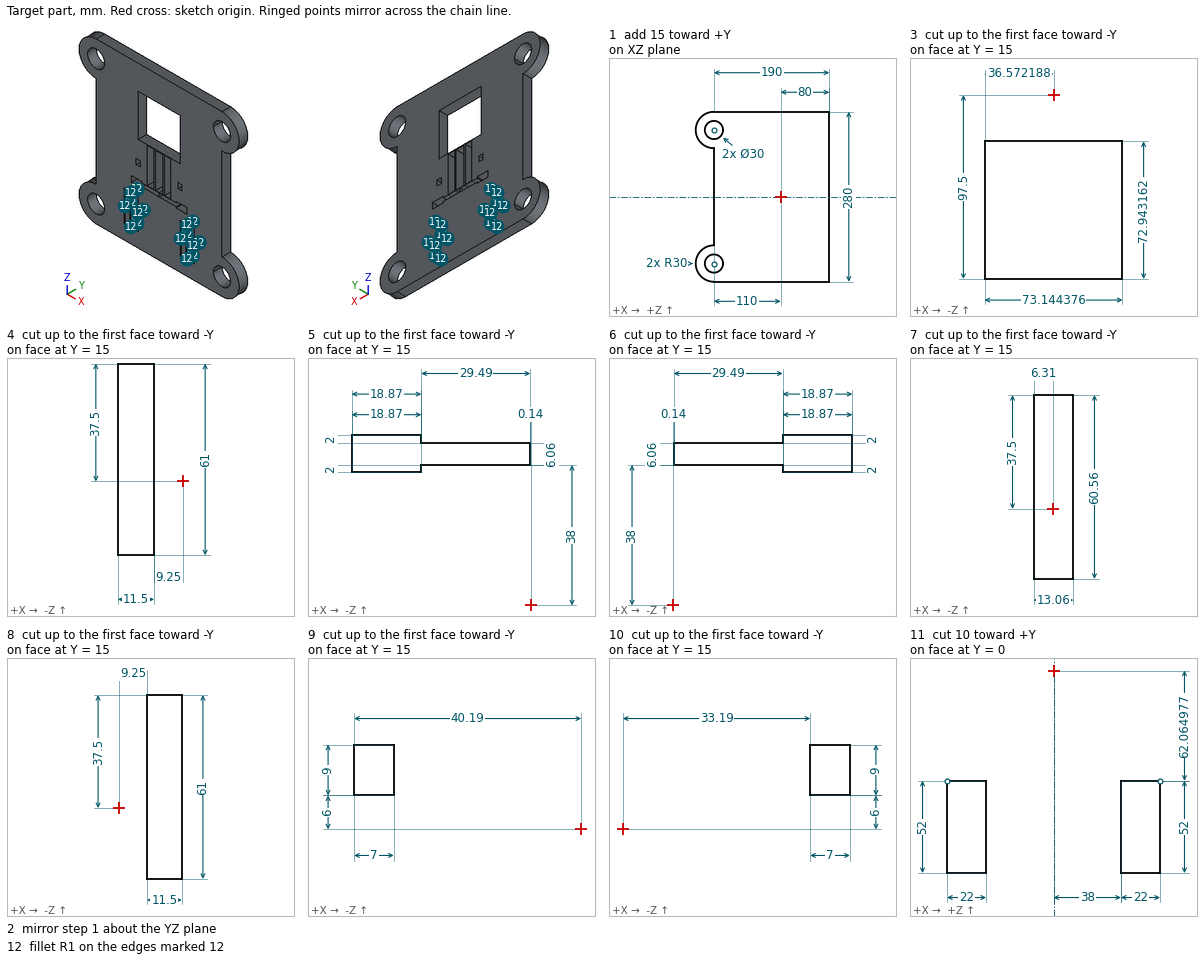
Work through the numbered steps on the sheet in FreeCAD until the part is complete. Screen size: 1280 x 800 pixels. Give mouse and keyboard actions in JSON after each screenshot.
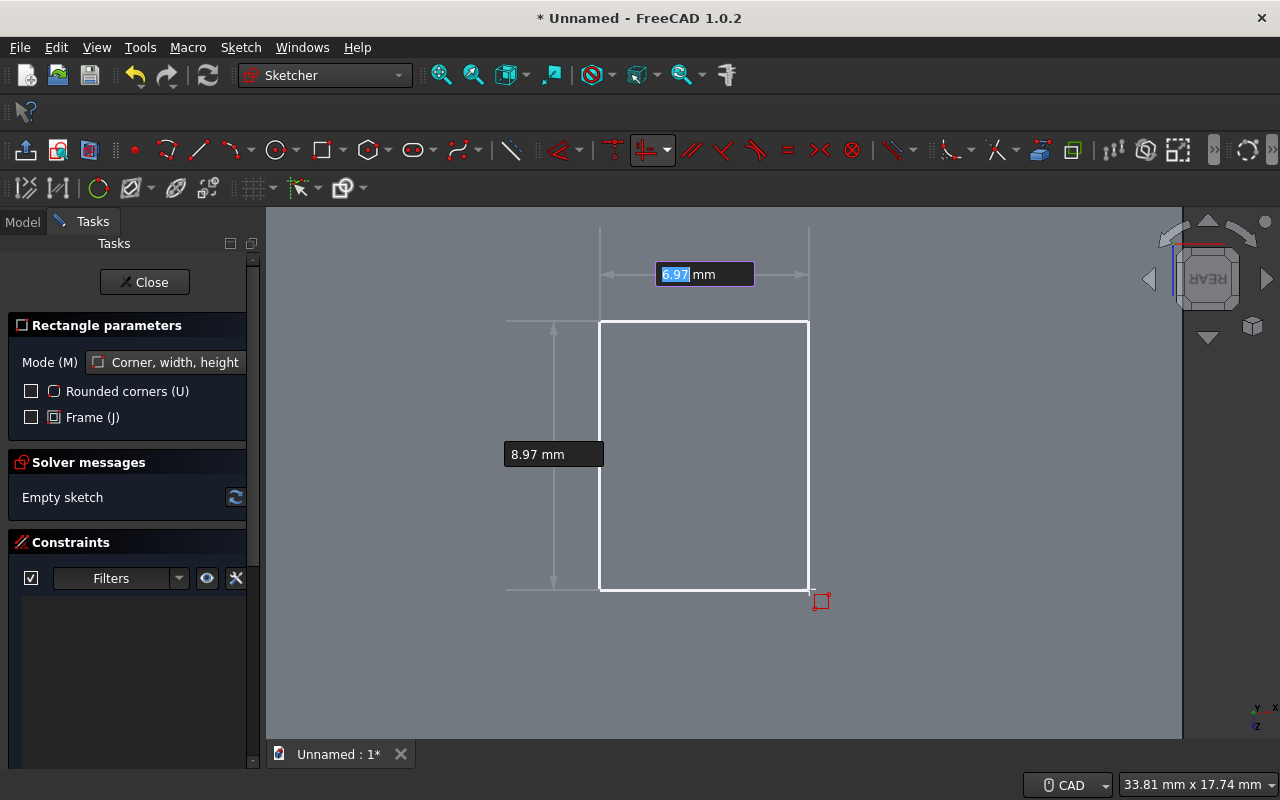
{"action": "type", "text": "7"}
{"action": "key", "text": "Tab"}
{"action": "type", "text": "9"}
{"action": "key", "text": "Return"}
{"action": "key", "text": "Escape"}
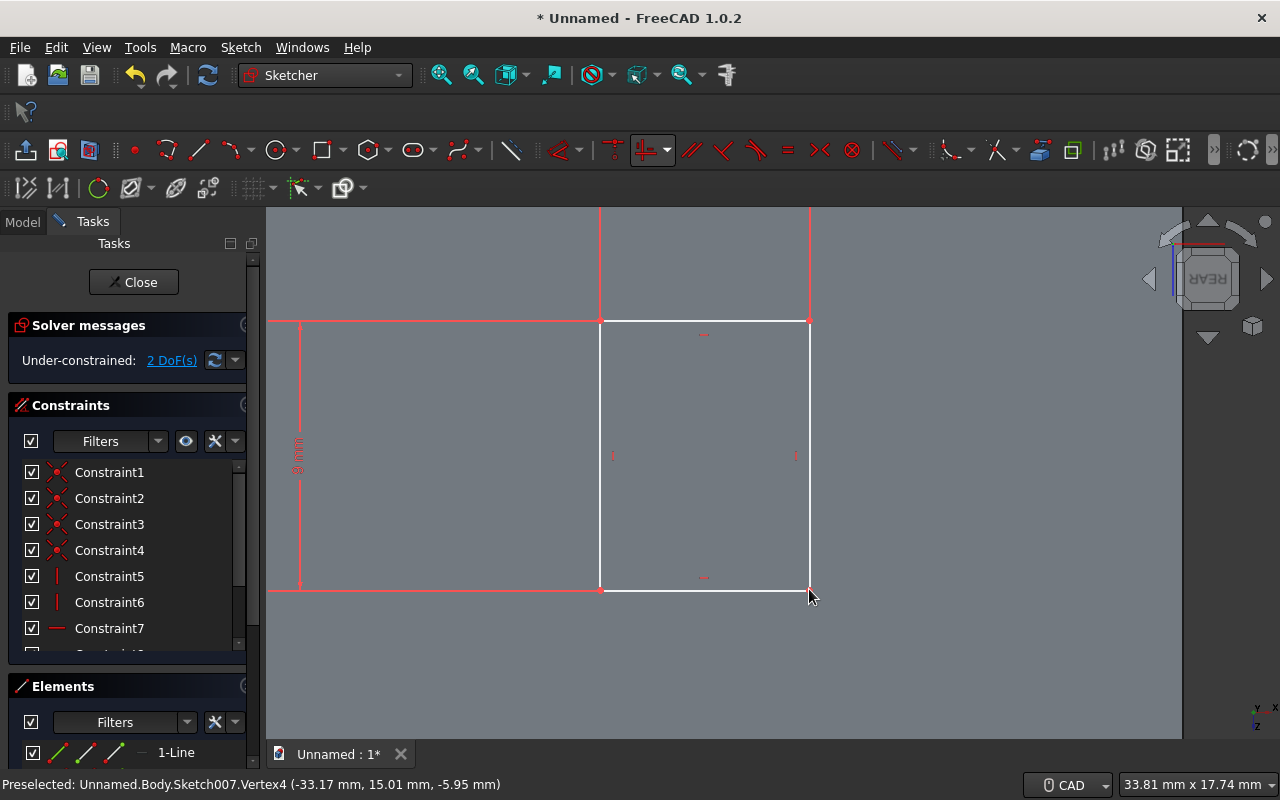
{"action": "left_click", "coordinate": [558, 150]}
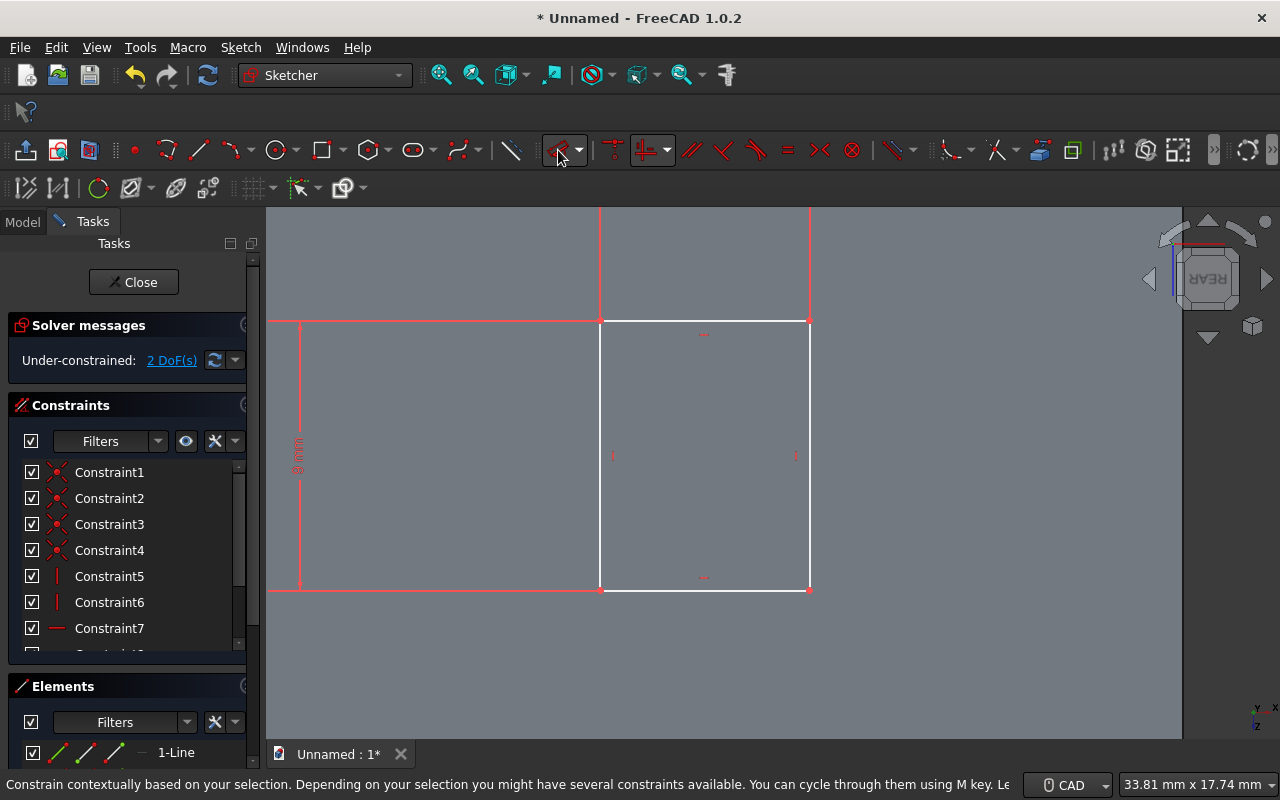
{"action": "left_click", "coordinate": [600, 591]}
{"action": "left_click", "coordinate": [566, 651]}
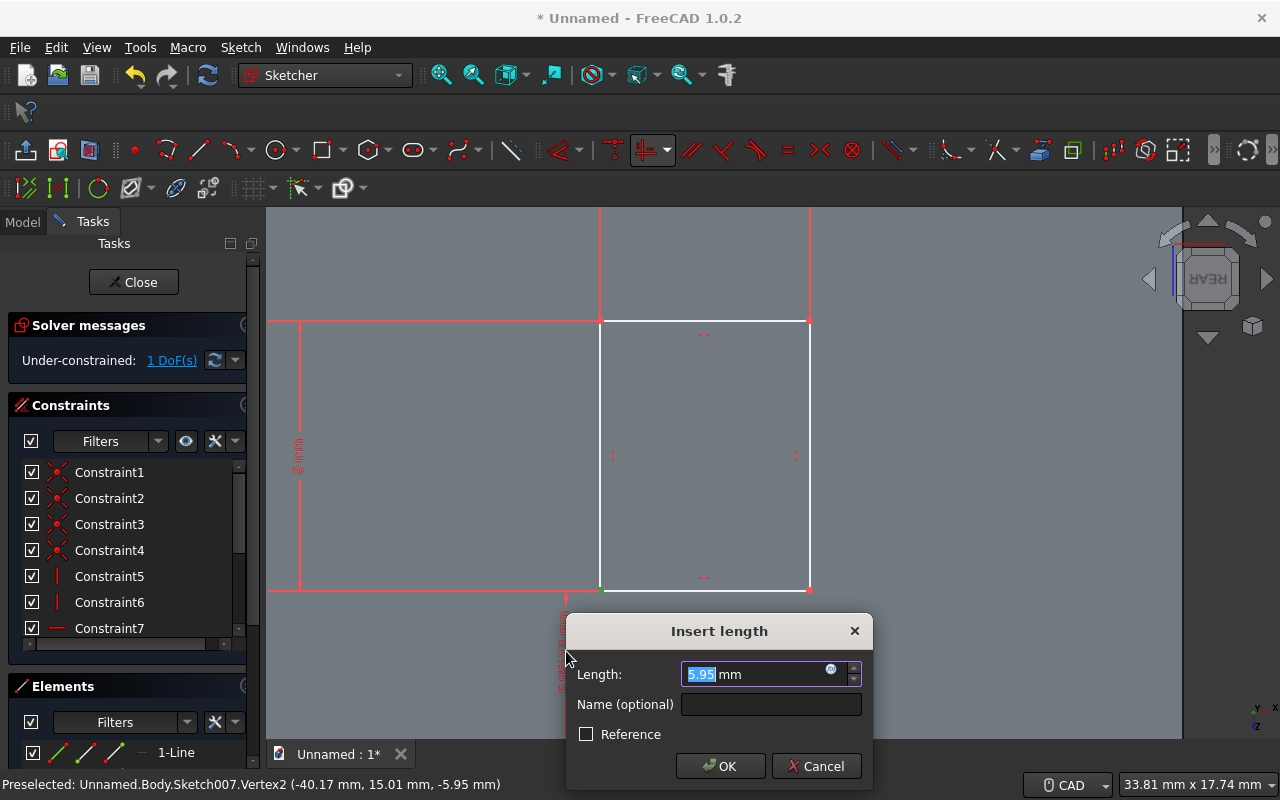
{"action": "type", "text": "6"}
{"action": "key", "text": "Return"}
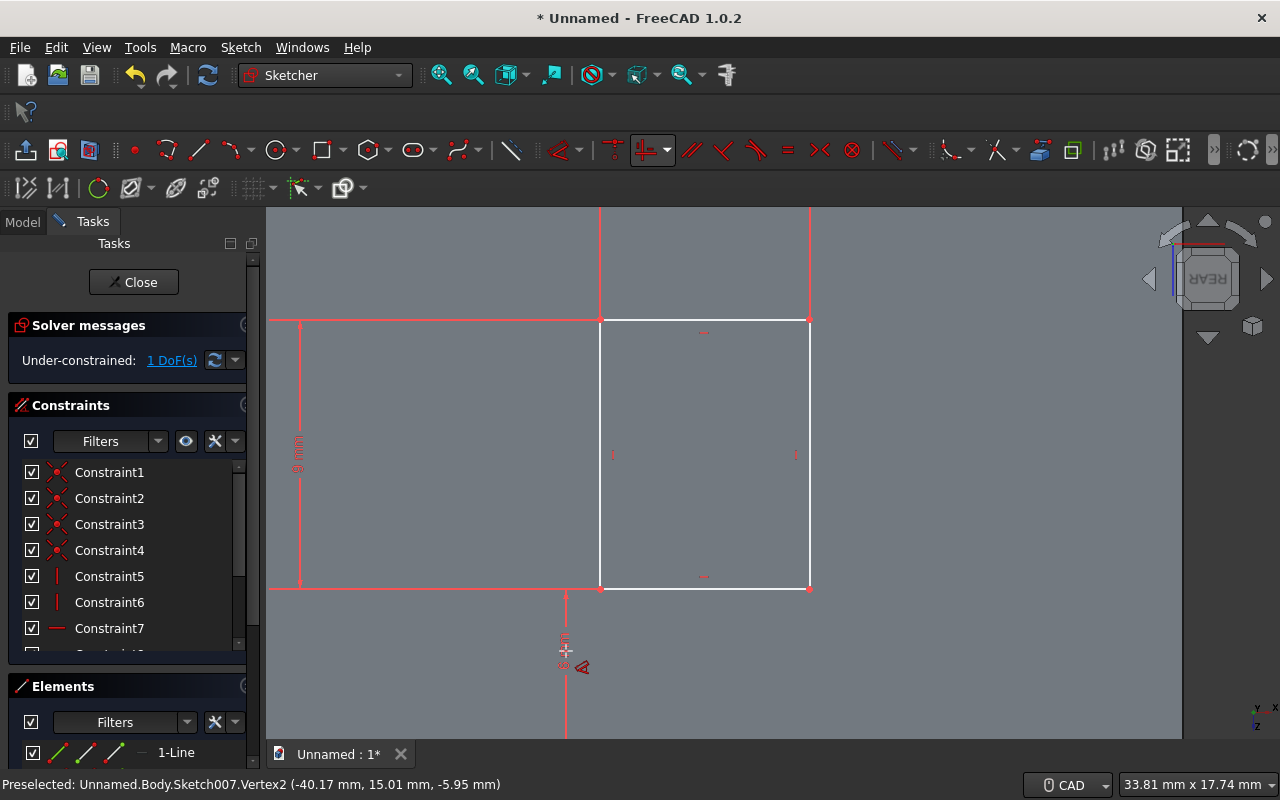
{"action": "left_click", "coordinate": [600, 320]}
{"action": "left_click", "coordinate": [858, 286]}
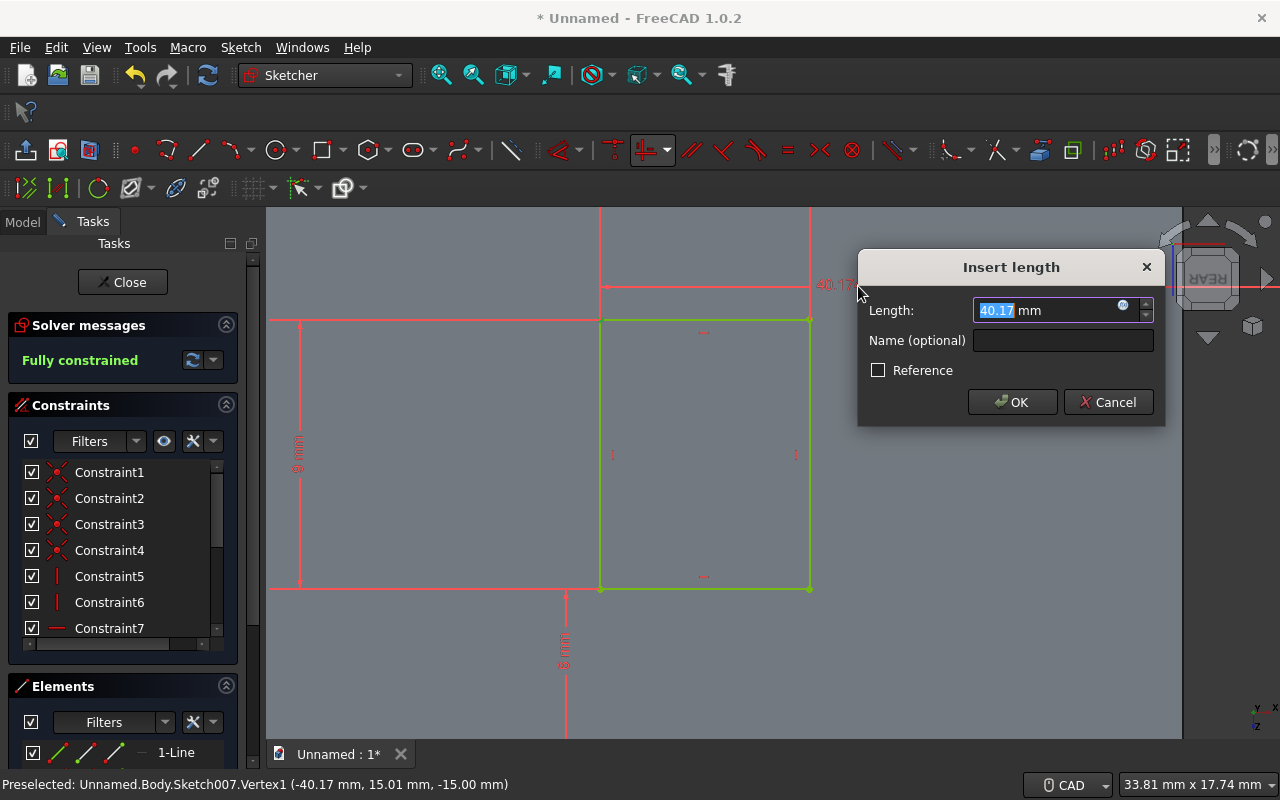
{"action": "type", "text": "40.19"}
{"action": "key", "text": "Return"}
{"action": "key", "text": "Escape"}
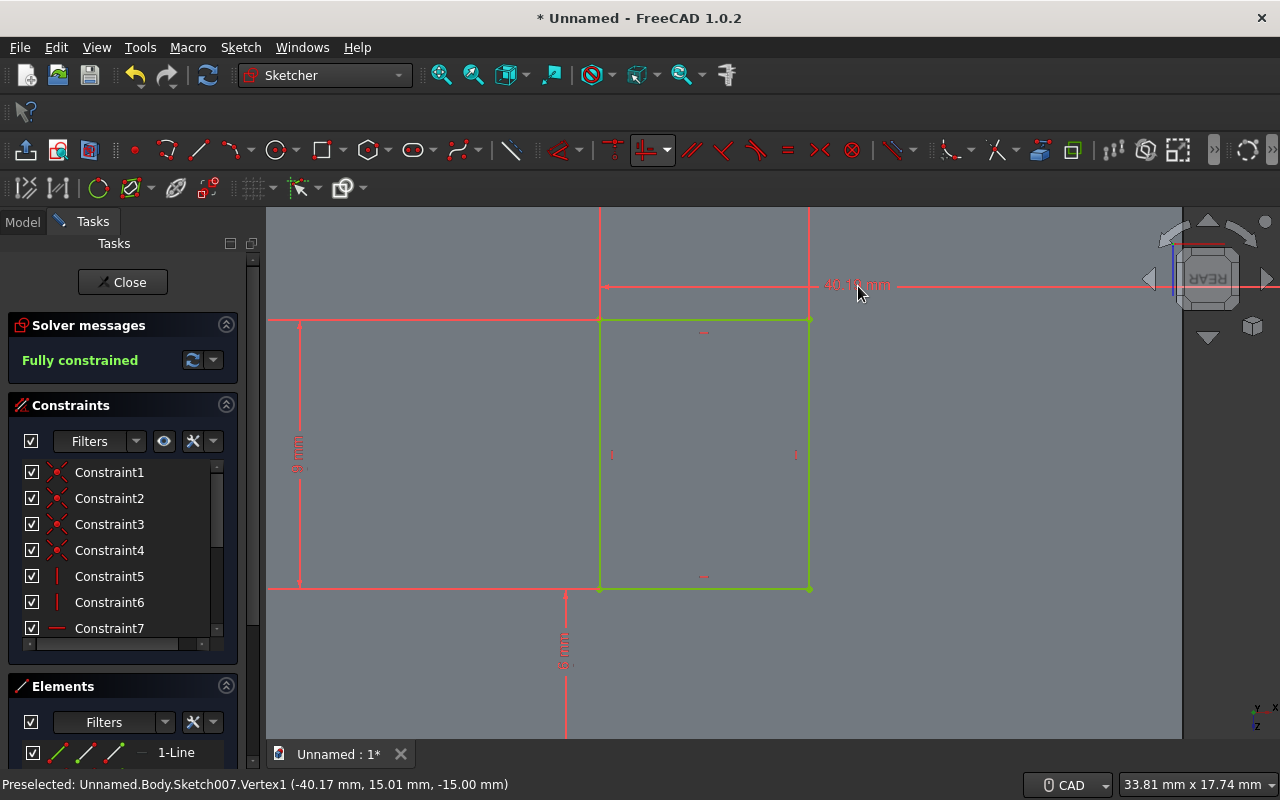
{"action": "left_click", "coordinate": [123, 282]}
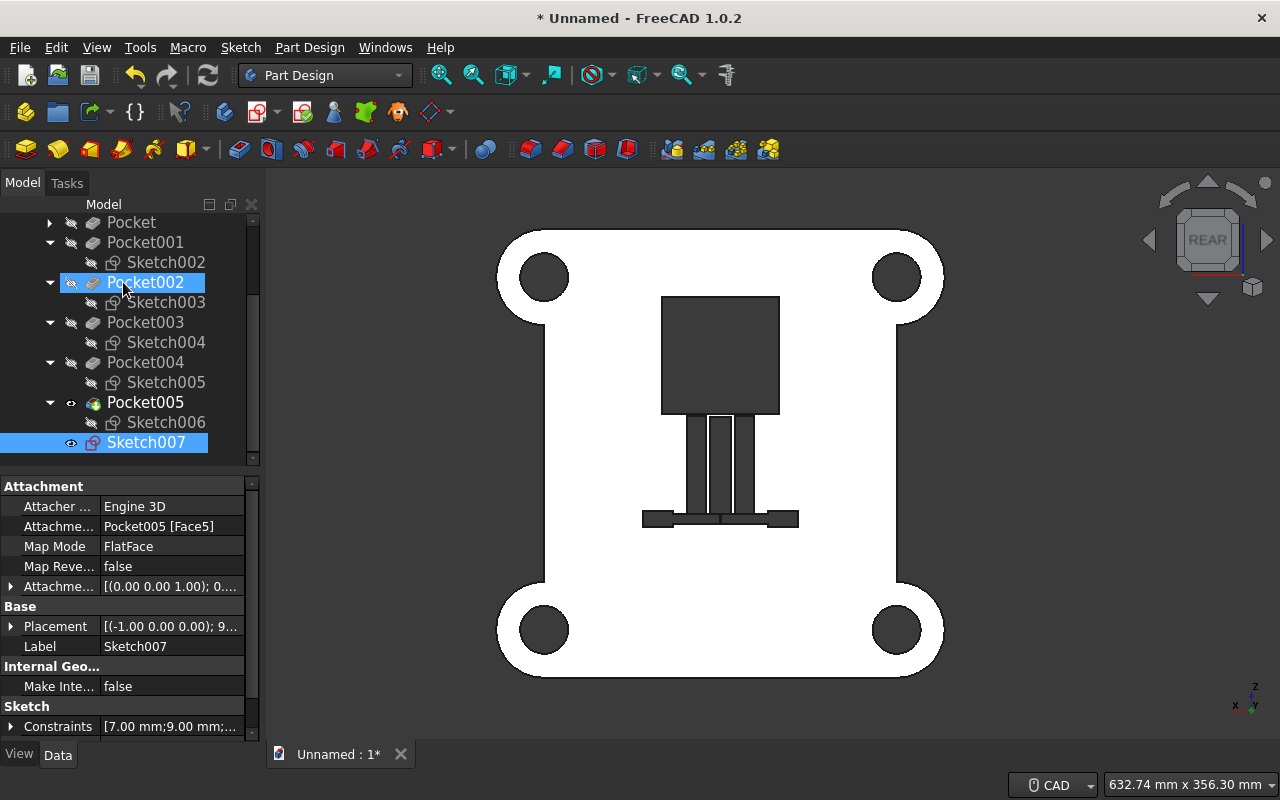
{"action": "left_click", "coordinate": [240, 150]}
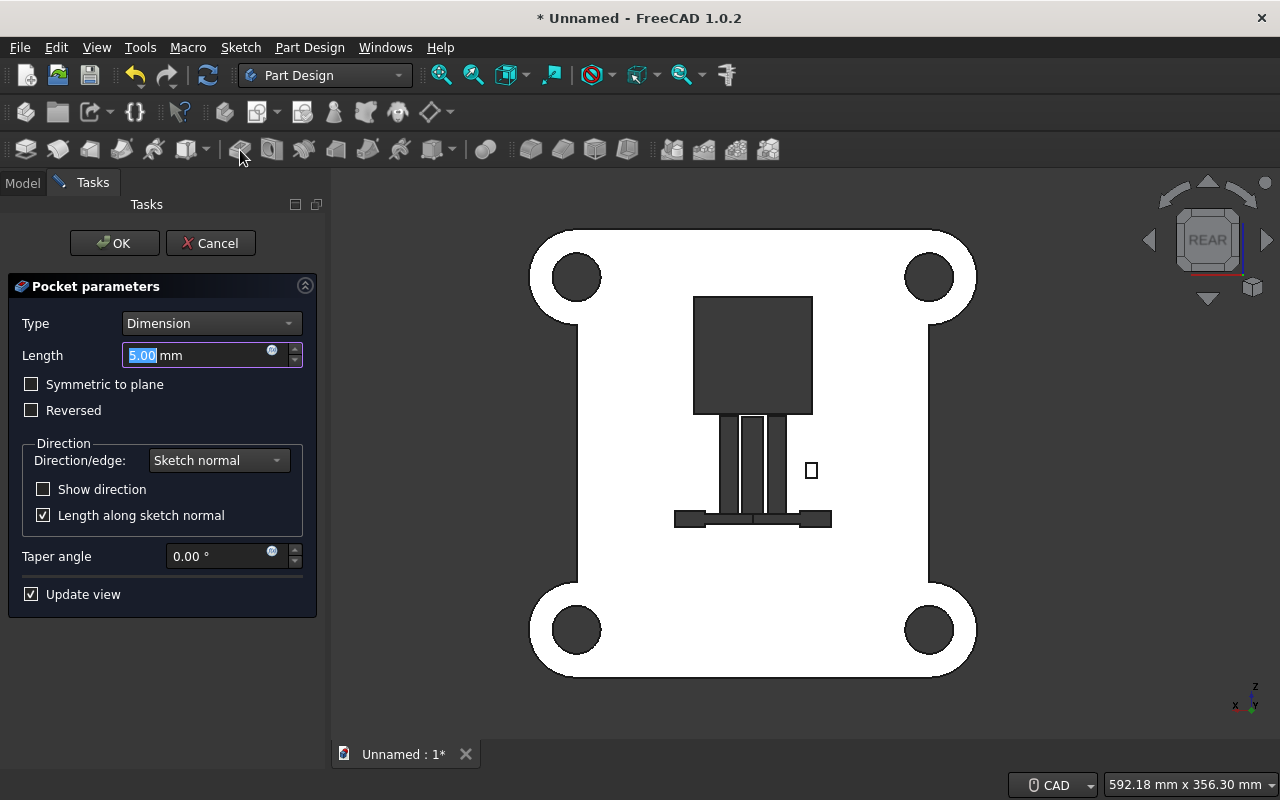
{"action": "left_click", "coordinate": [212, 324]}